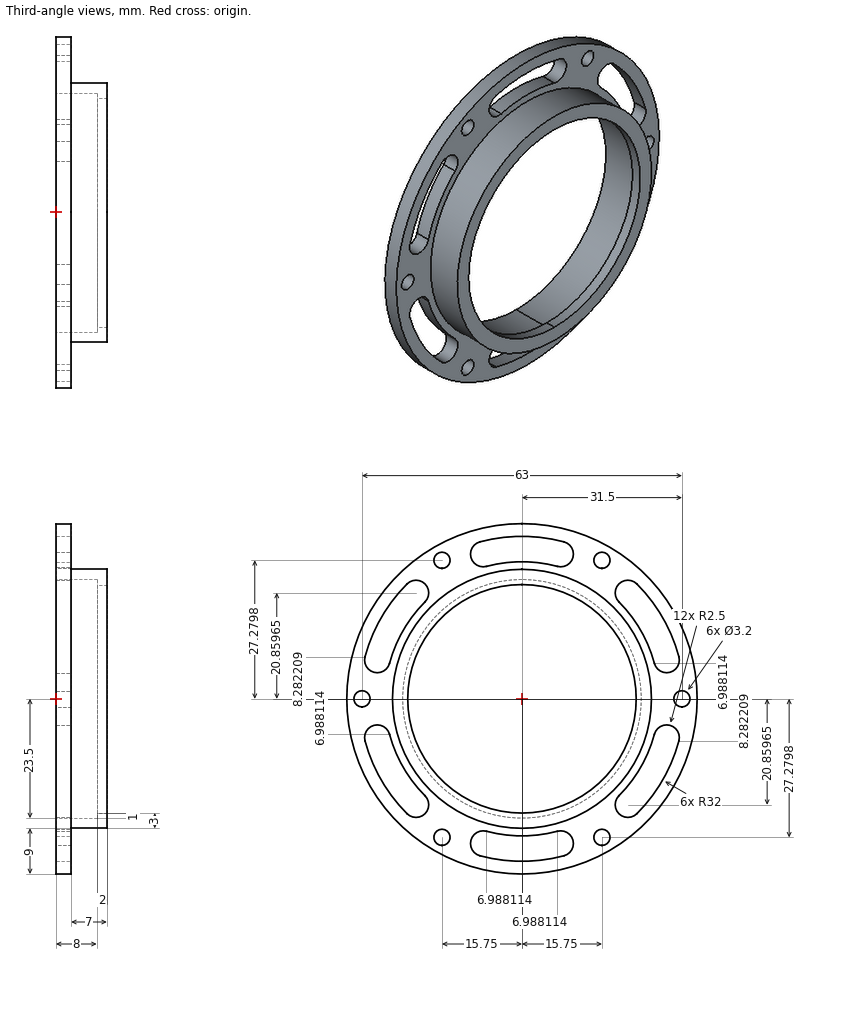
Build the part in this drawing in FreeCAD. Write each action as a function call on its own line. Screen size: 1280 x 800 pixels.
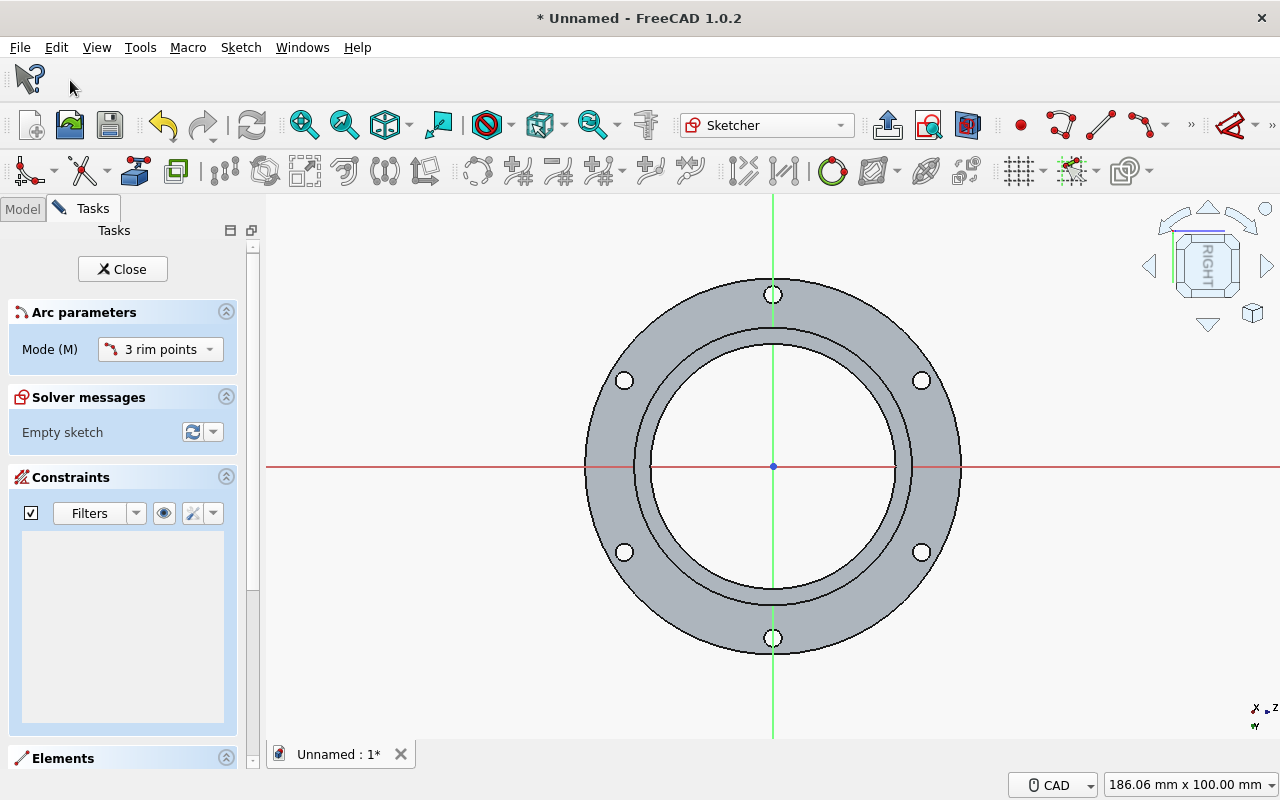
click(669, 571)
click(650, 590)
click(650, 571)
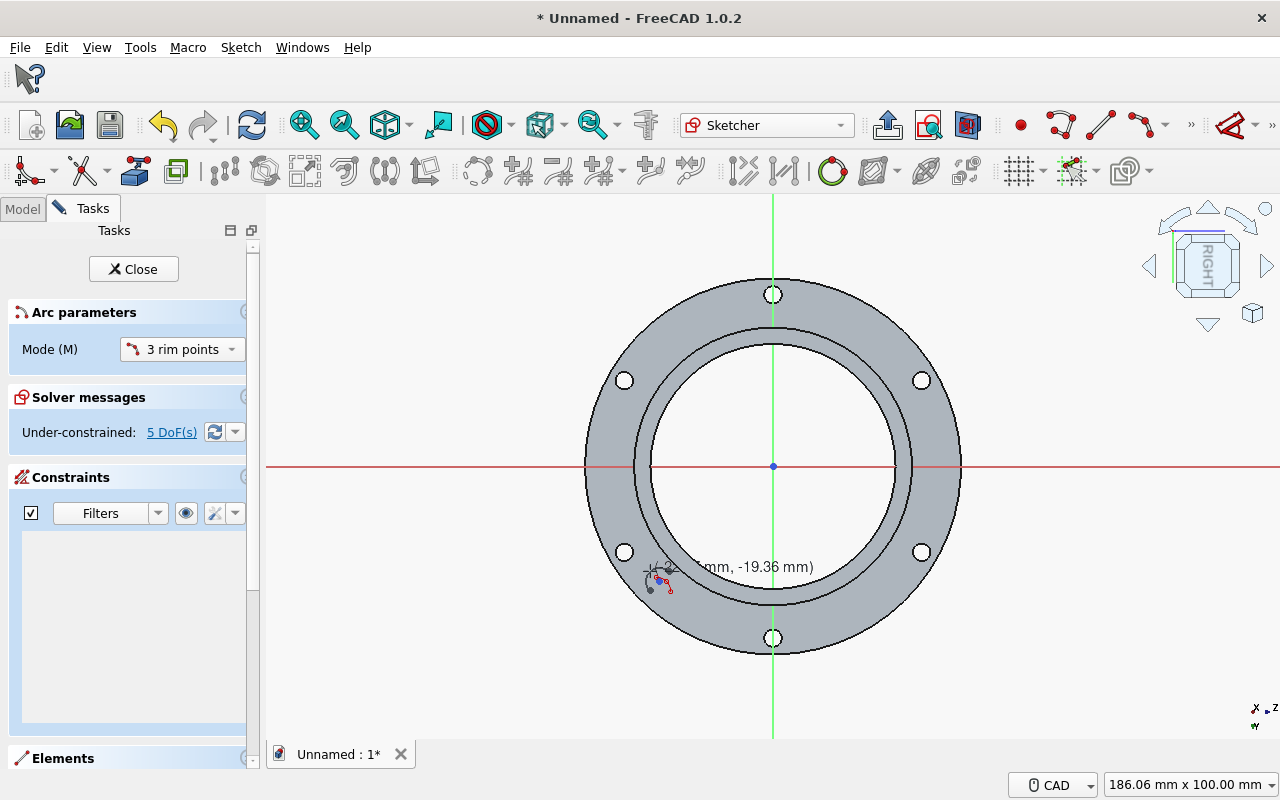
click(650, 591)
click(728, 635)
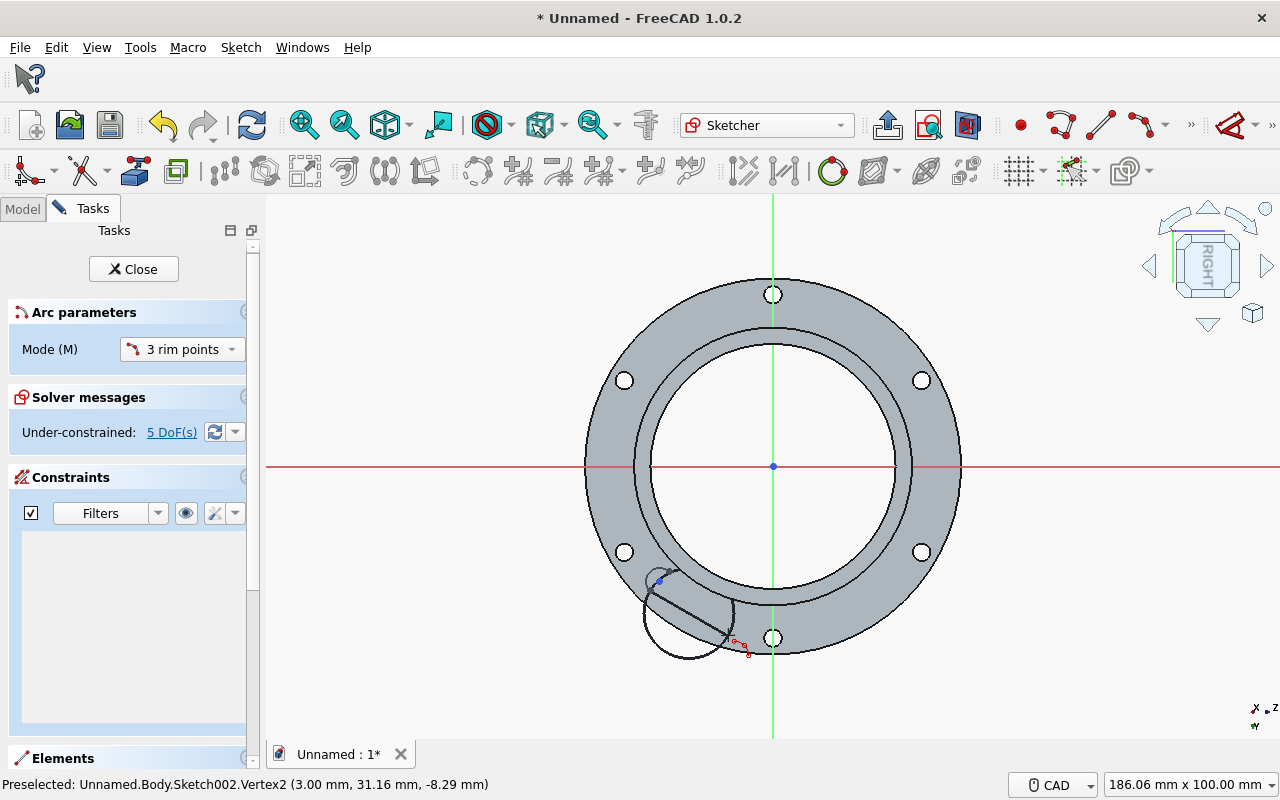
scroll(686, 618, up, 5)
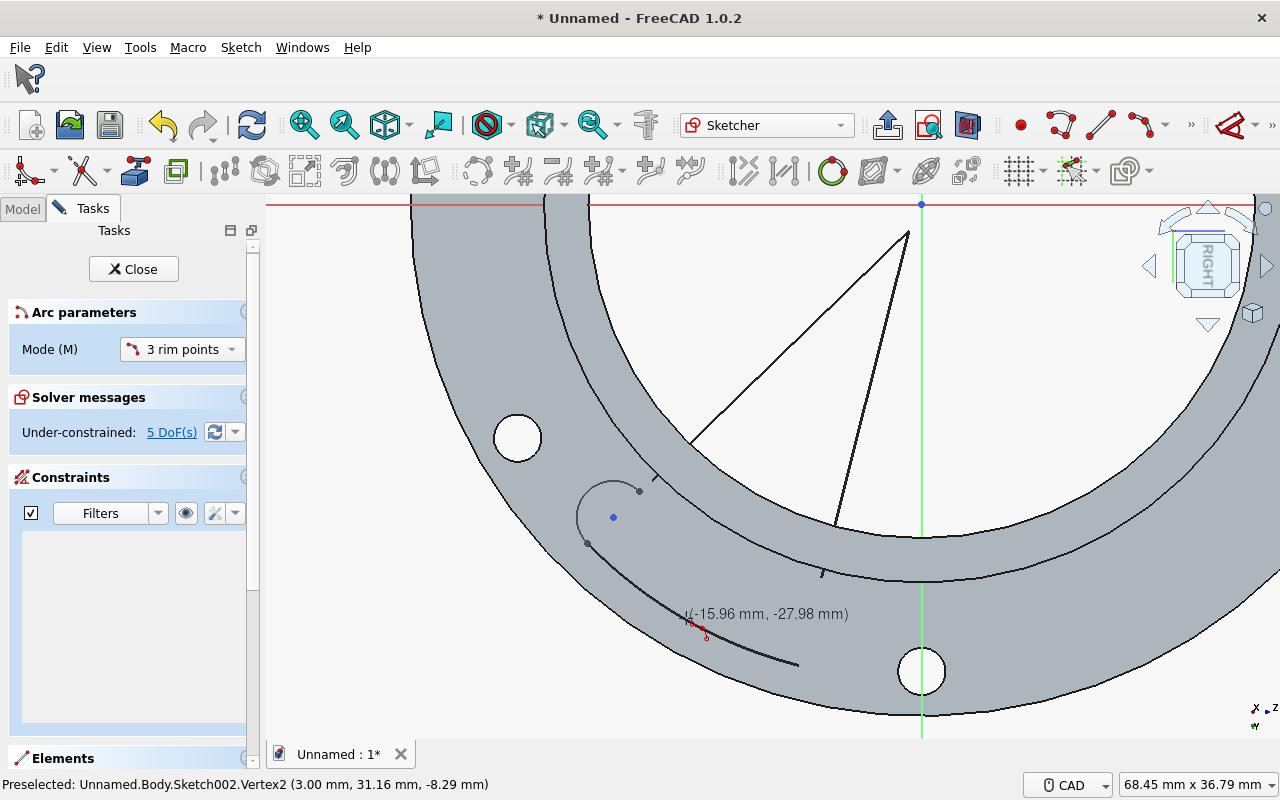
click(685, 615)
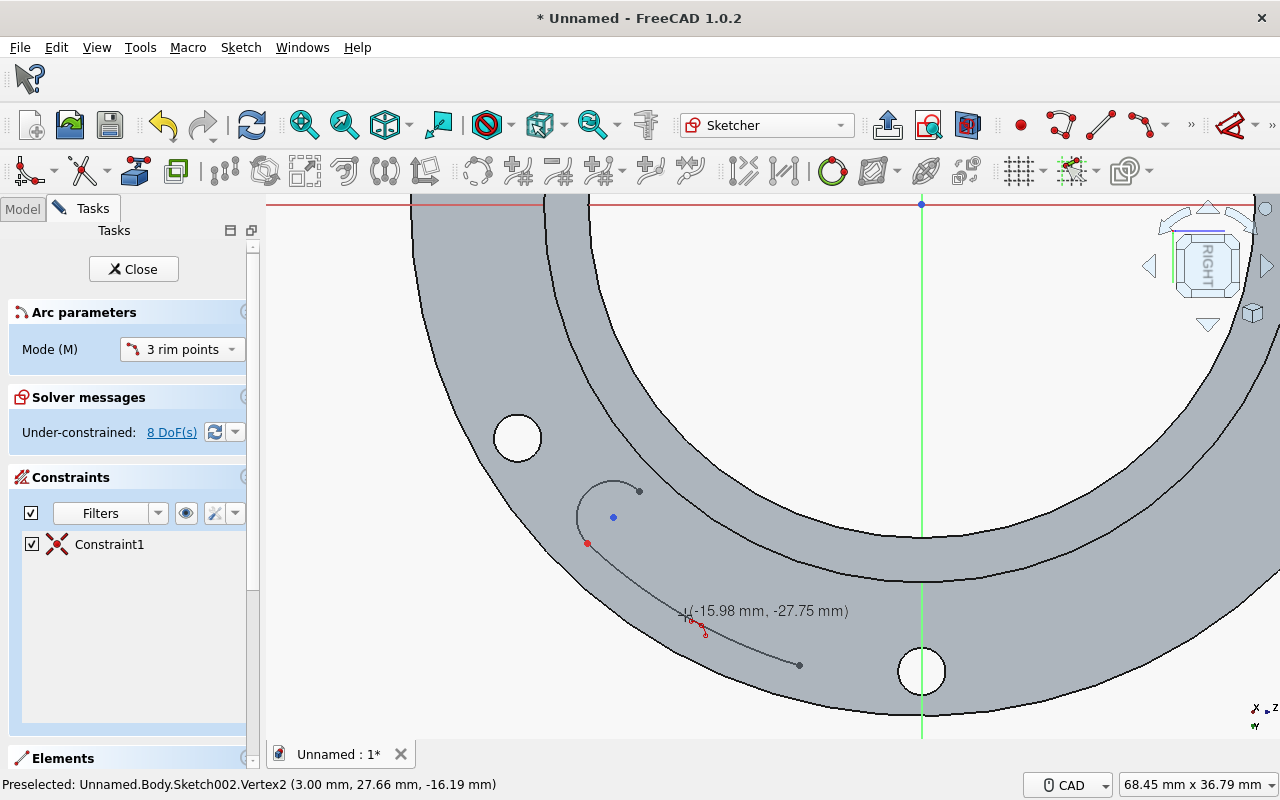
click(799, 666)
click(818, 591)
click(844, 637)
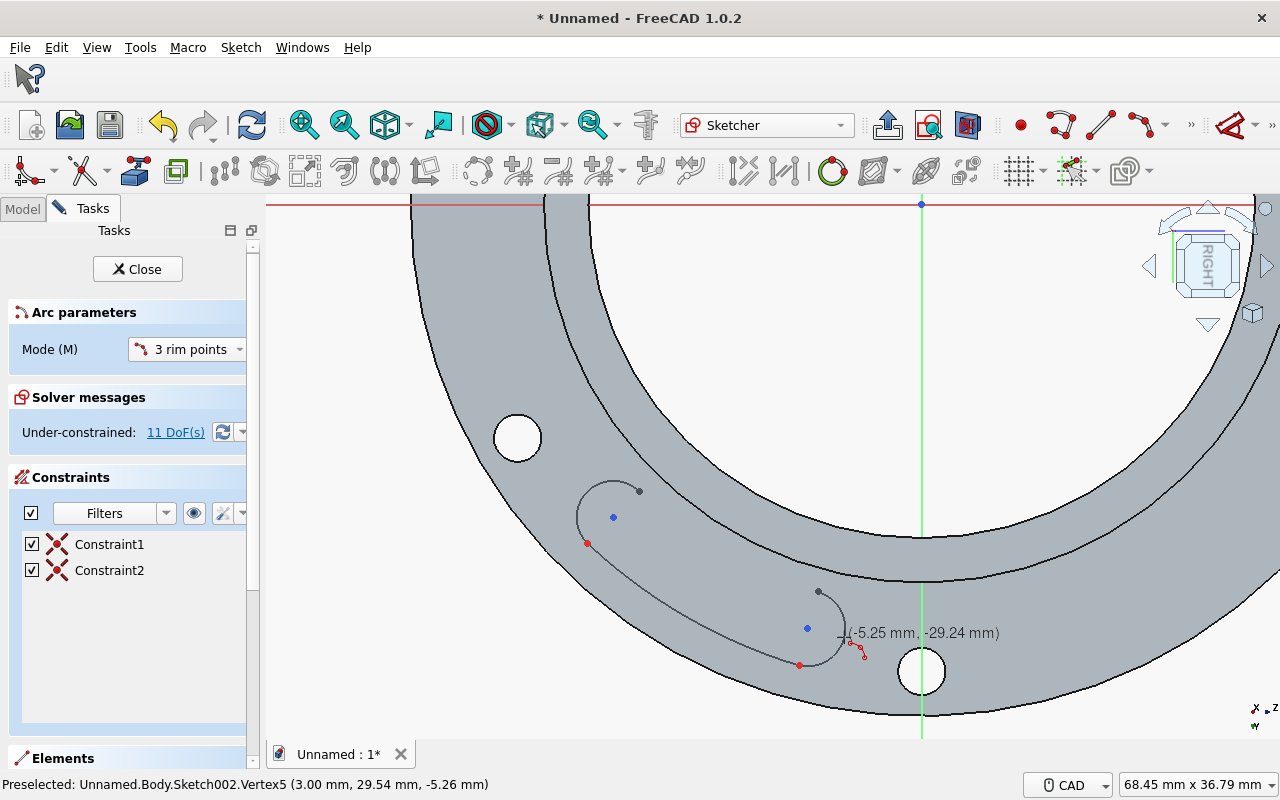
click(818, 592)
click(639, 492)
click(722, 551)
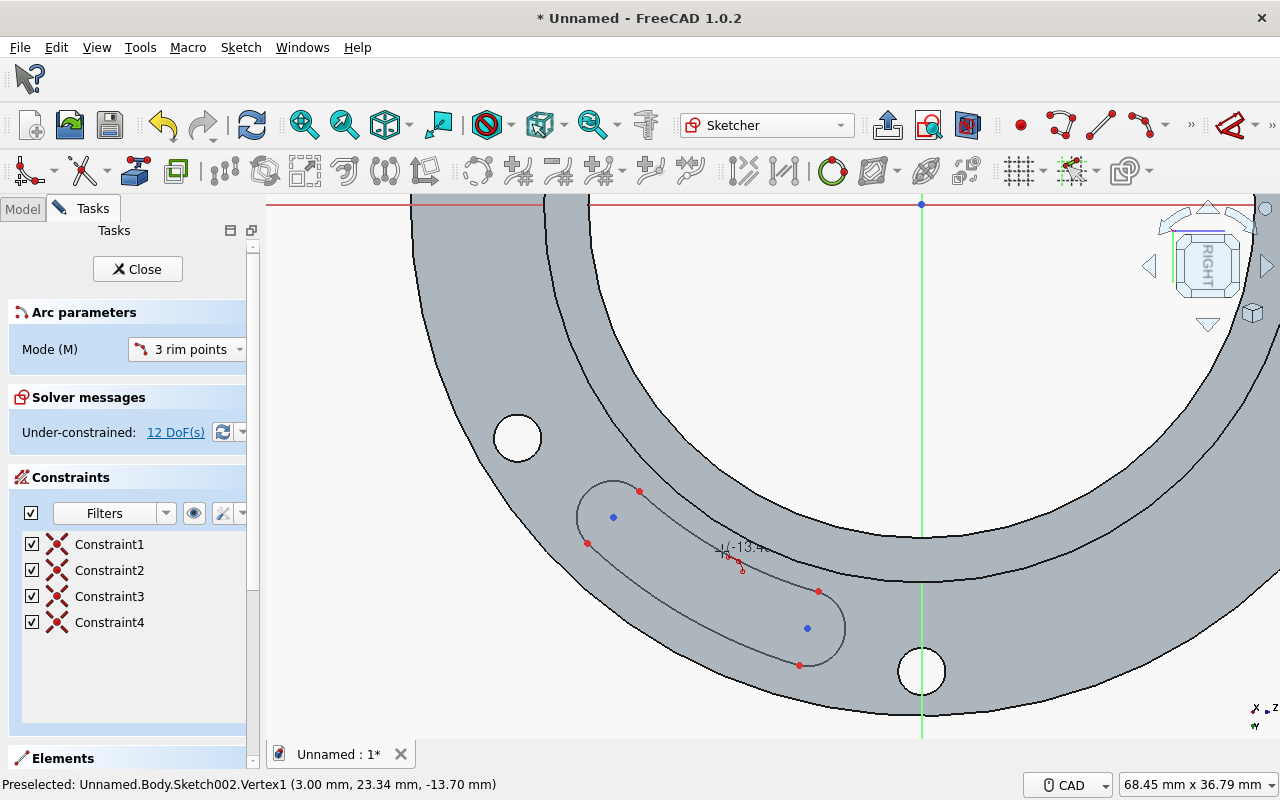
click(535, 308)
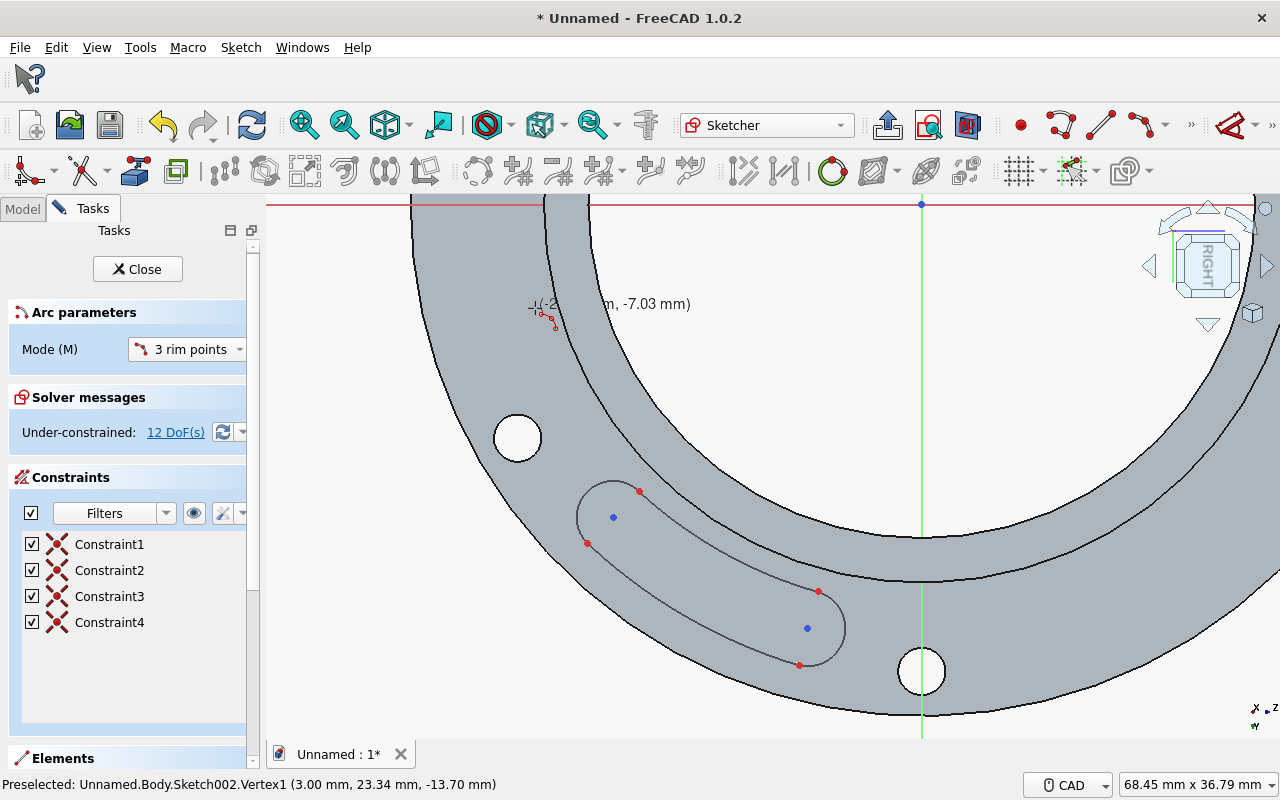
scroll(578, 619, down, 5)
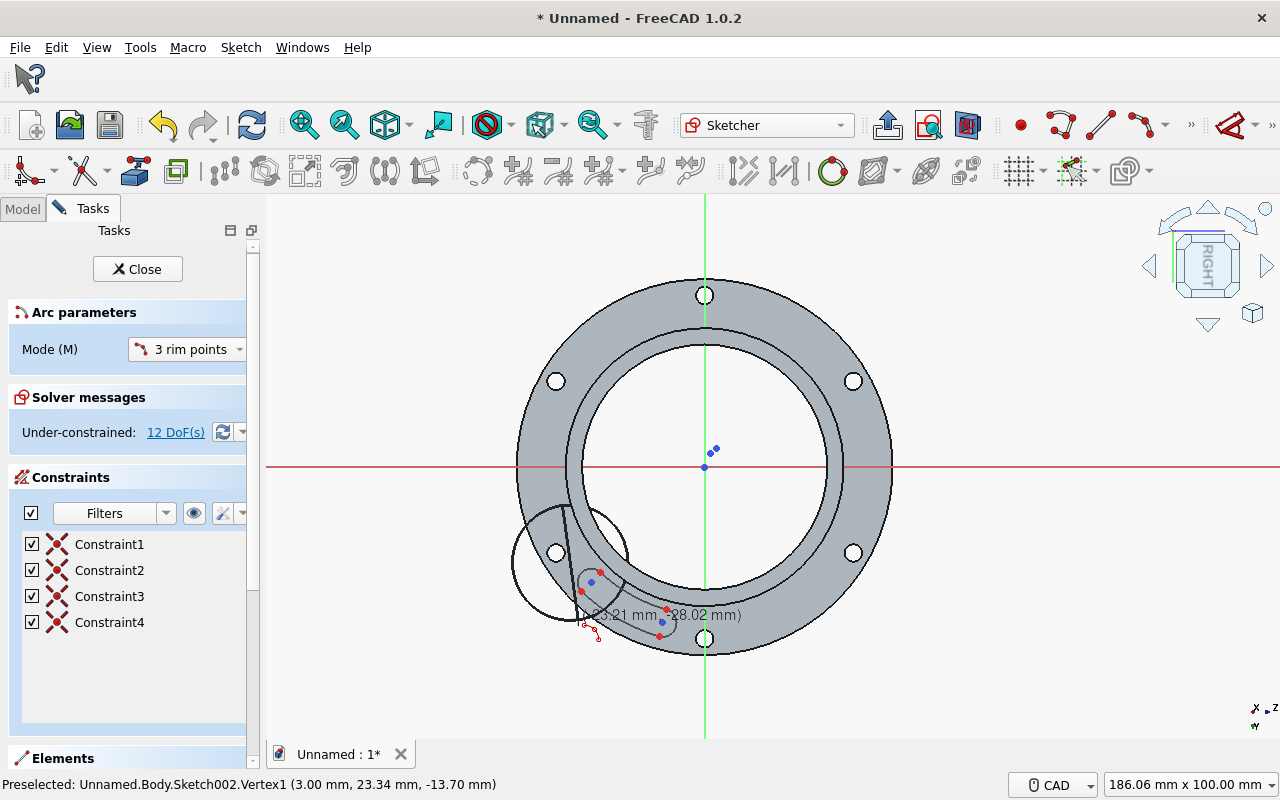
click(563, 429)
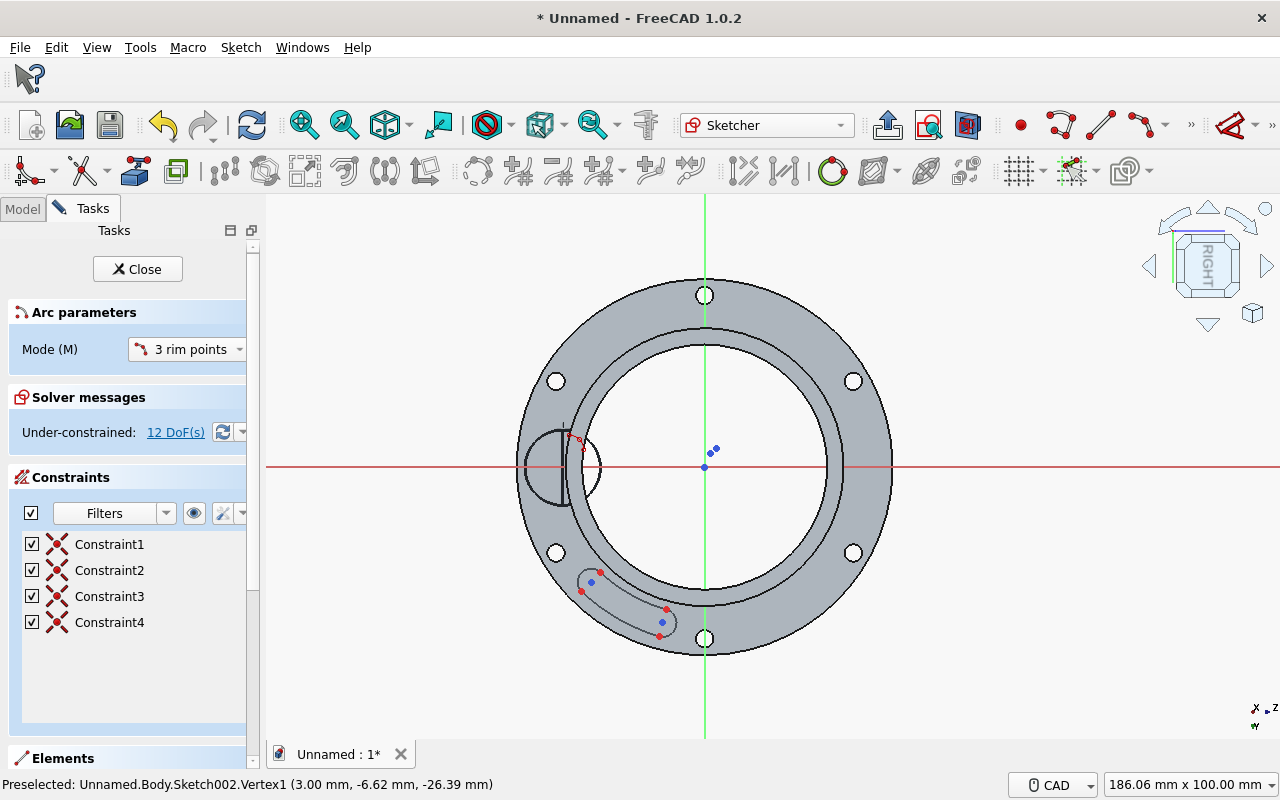
scroll(558, 459, up, 6)